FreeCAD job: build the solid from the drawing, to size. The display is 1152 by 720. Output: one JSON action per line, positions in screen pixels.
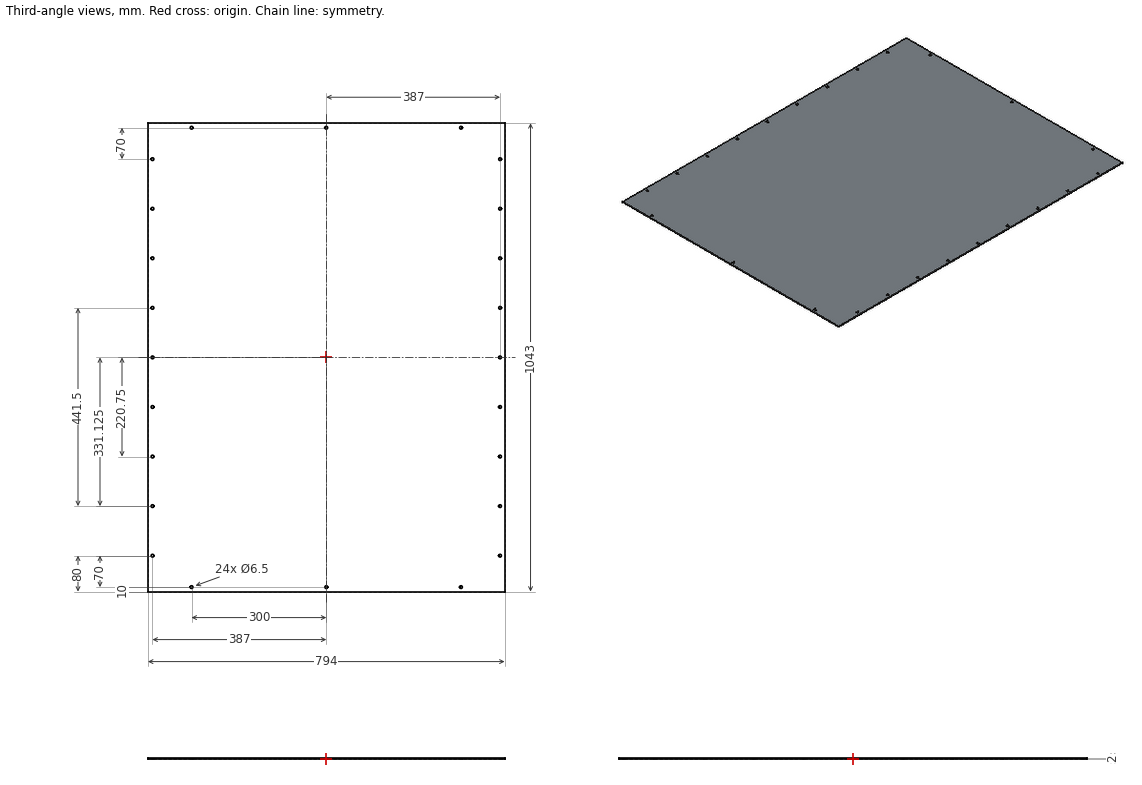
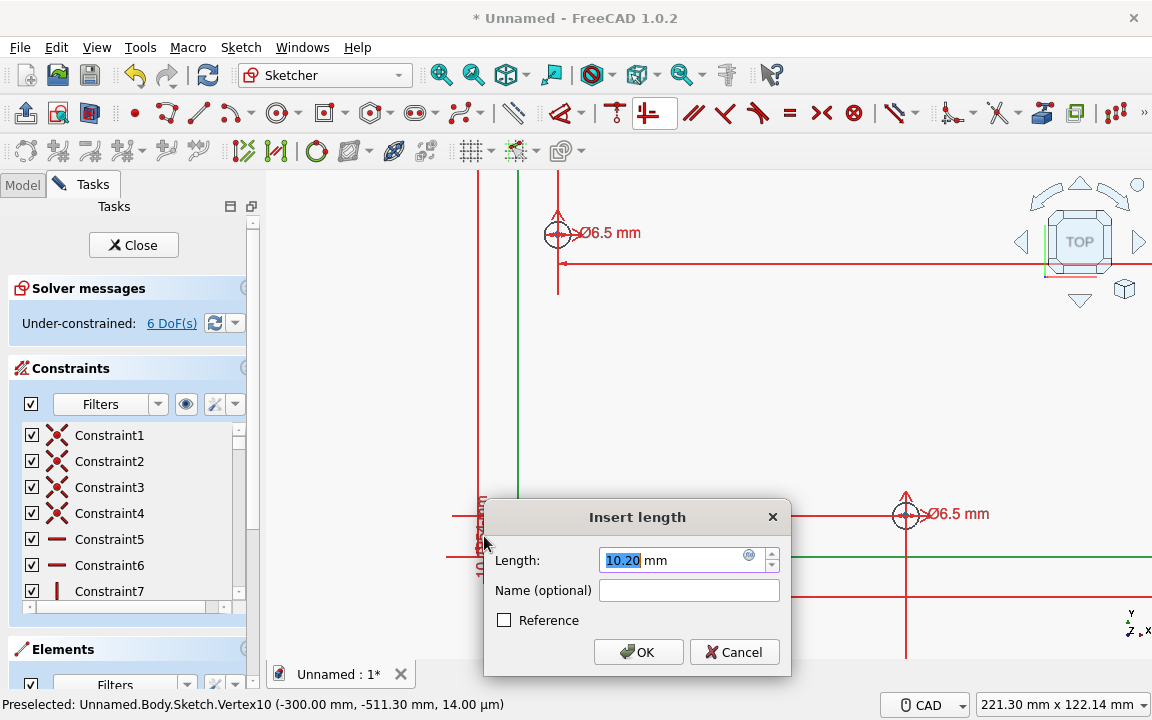
{"action": "type", "text": "10"}
{"action": "key", "text": "Return"}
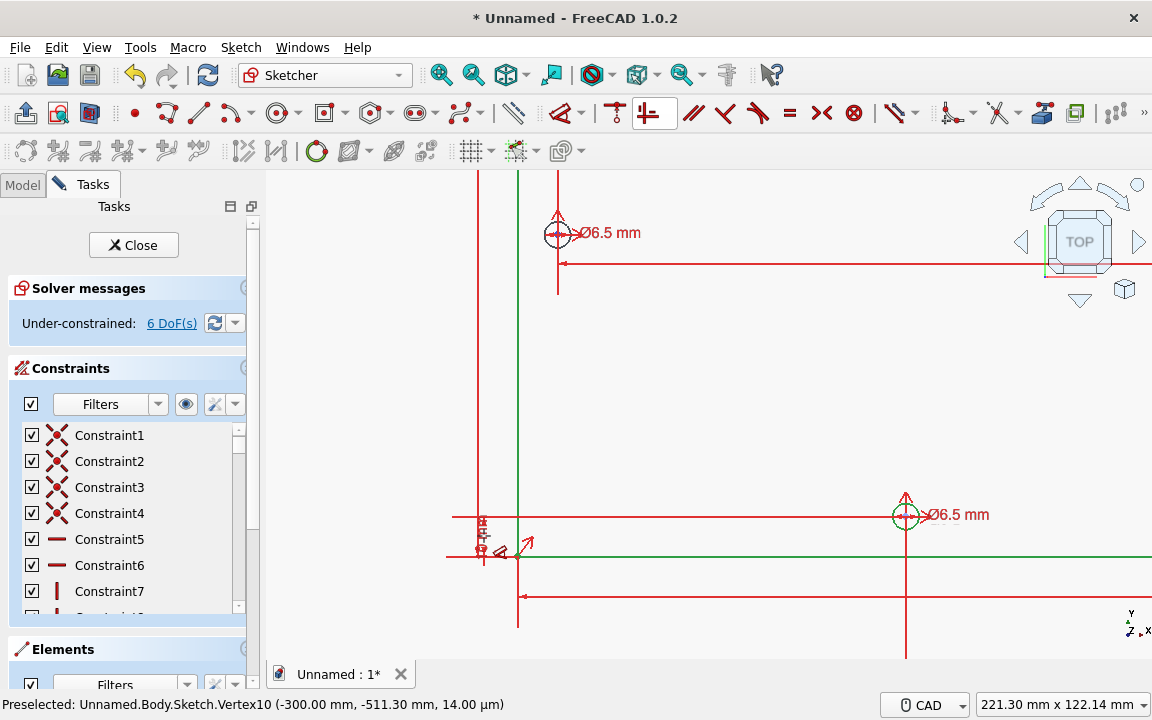
{"action": "scroll", "coordinate": [523, 571], "scroll_direction": "down", "scroll_amount": 13}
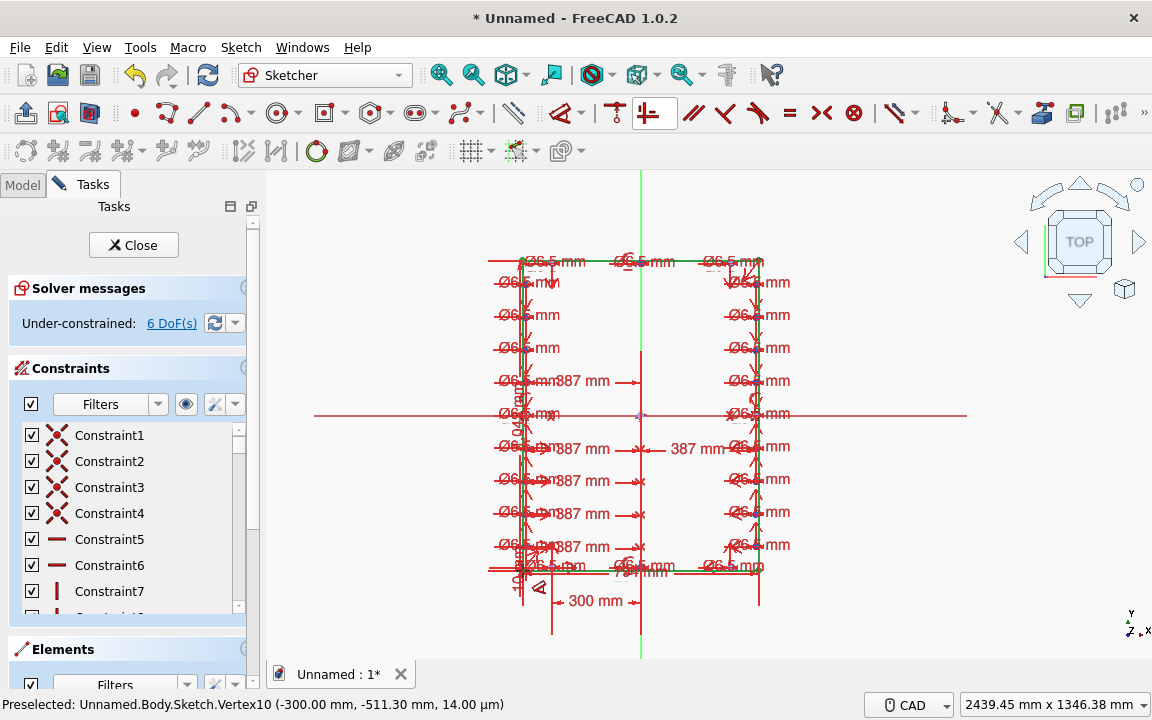
{"action": "scroll", "coordinate": [523, 571], "scroll_direction": "up", "scroll_amount": 3}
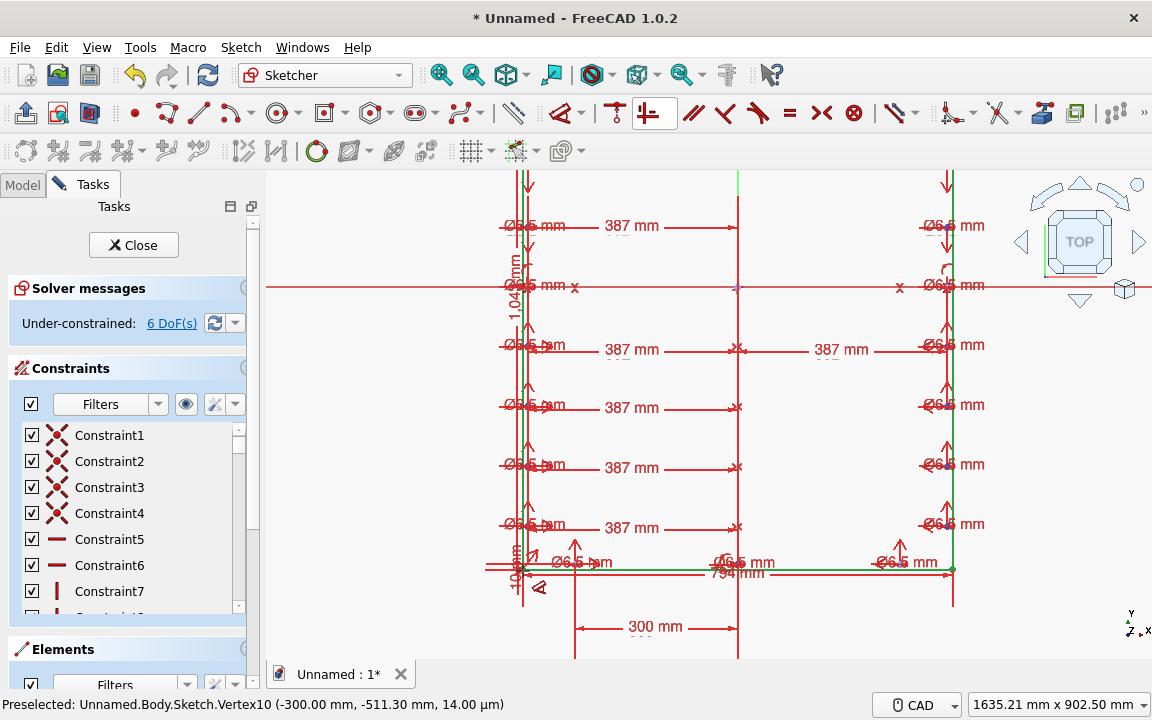
{"action": "left_click", "coordinate": [523, 570]}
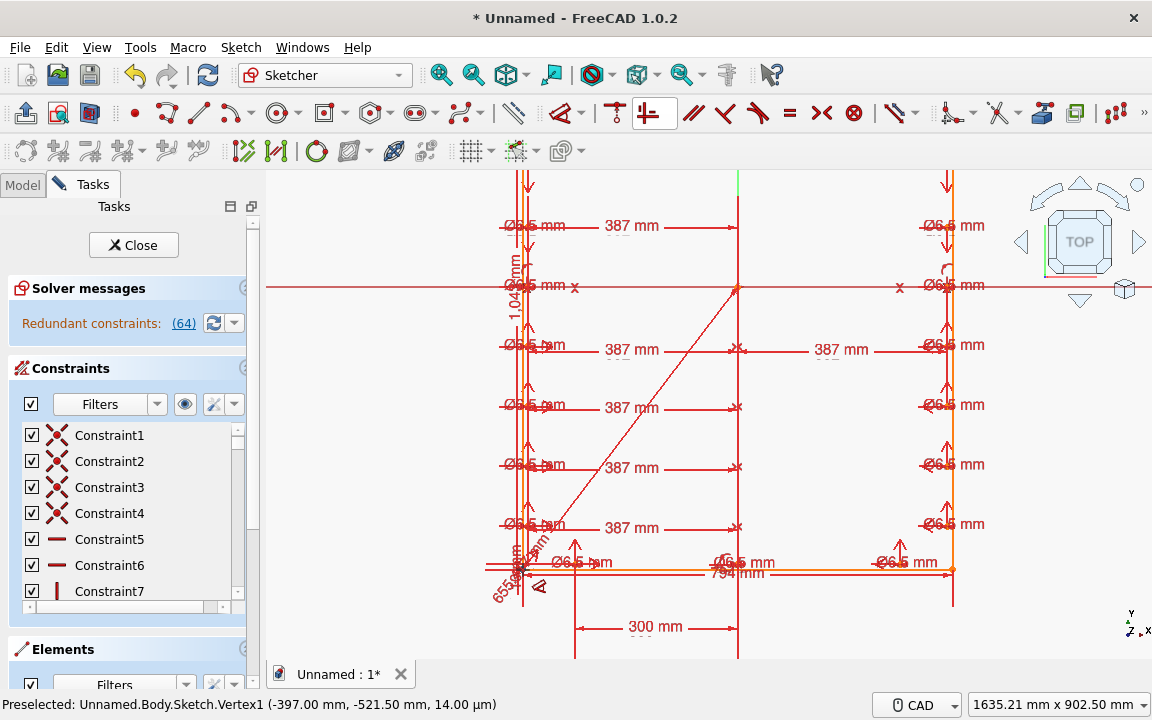
{"action": "left_click", "coordinate": [528, 526]}
{"action": "left_click", "coordinate": [489, 538]}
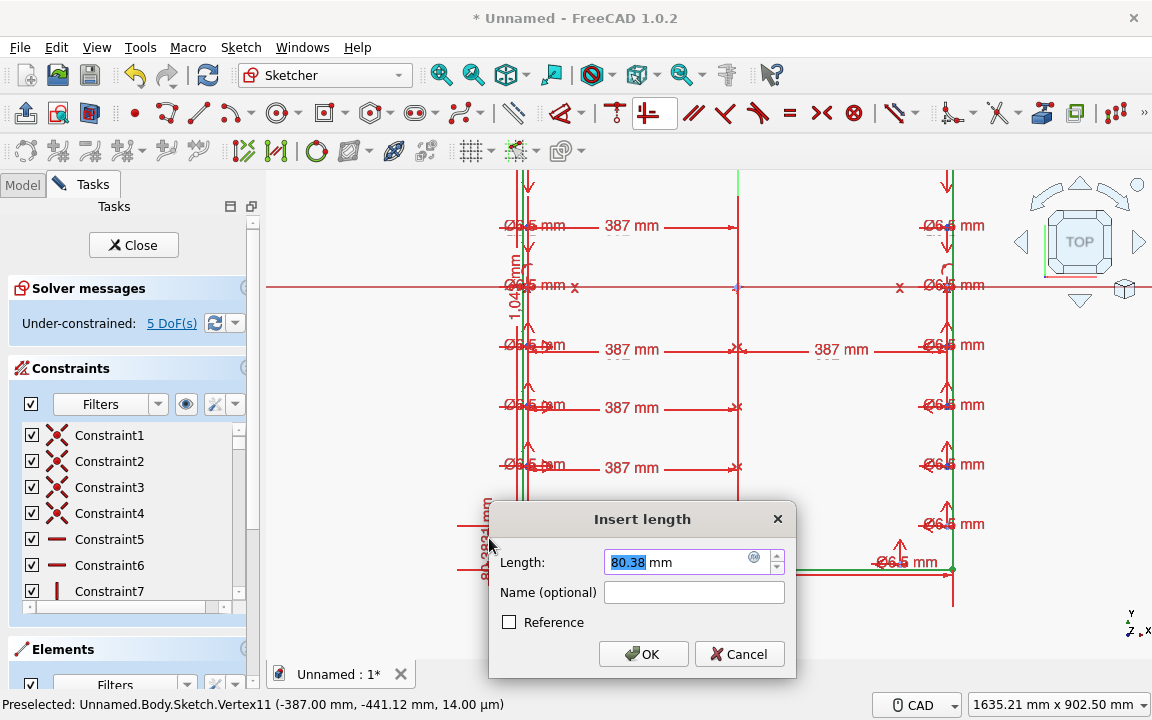
{"action": "type", "text": "80"}
{"action": "key", "text": "Return"}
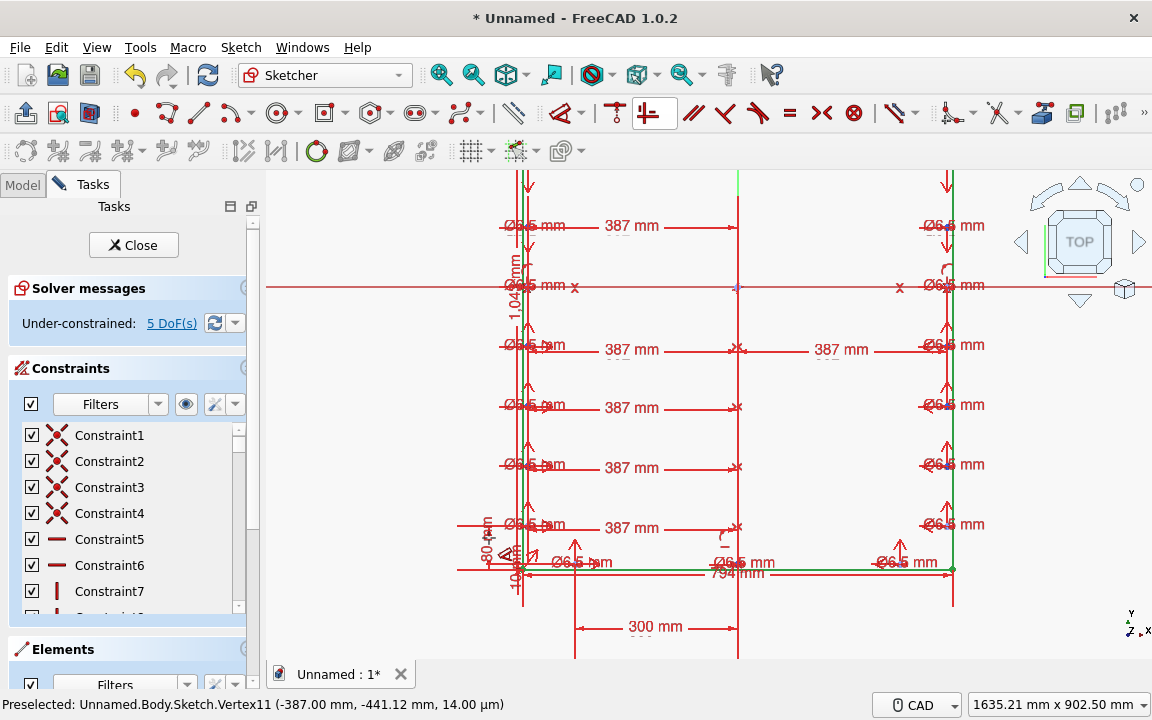
{"action": "left_click", "coordinate": [528, 526]}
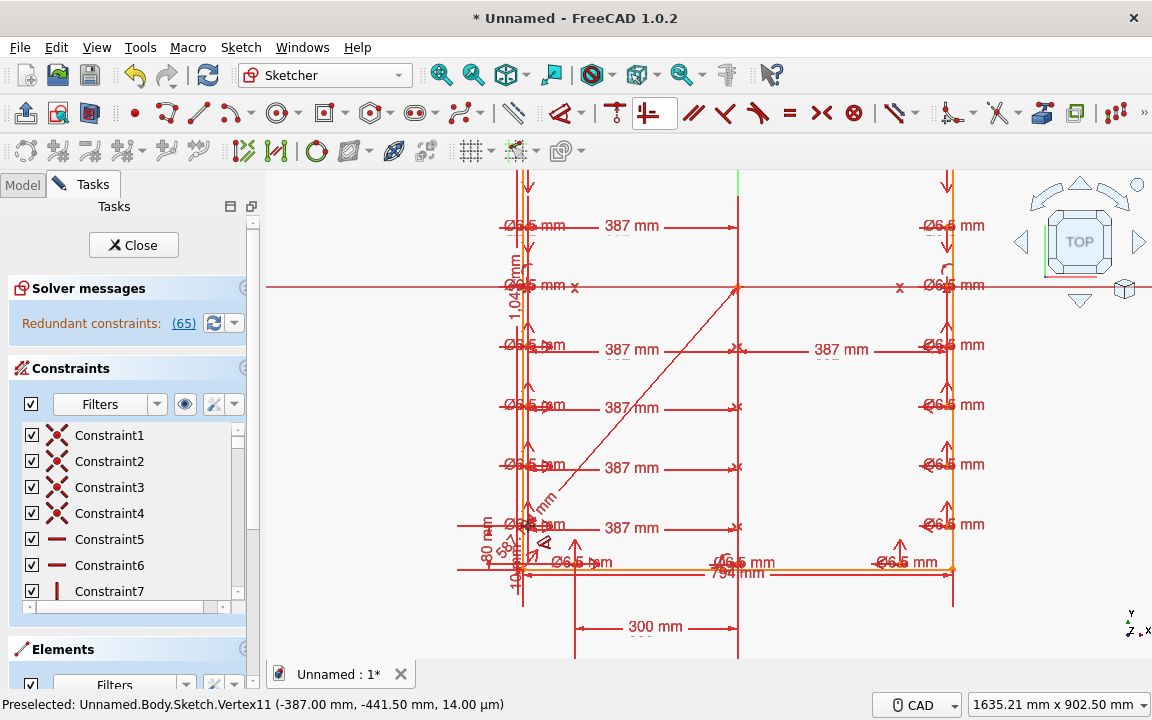
{"action": "left_click", "coordinate": [738, 565]}
{"action": "left_click", "coordinate": [772, 545]}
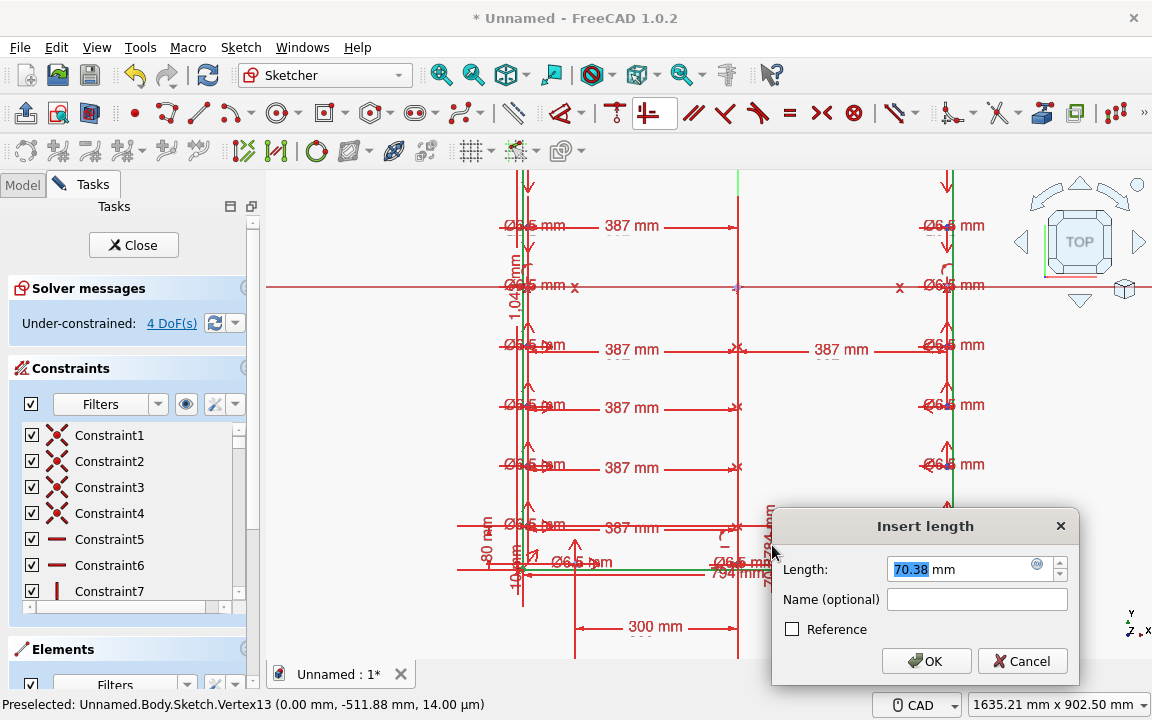
{"action": "type", "text": "70"}
{"action": "key", "text": "Return"}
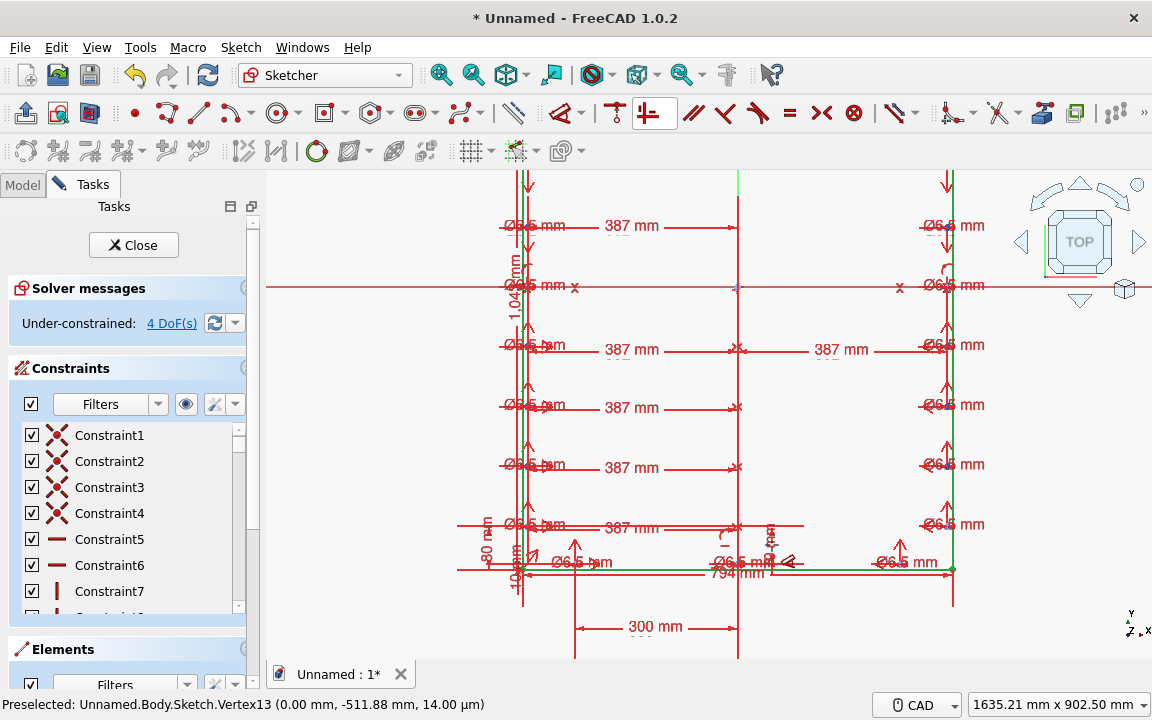
{"action": "scroll", "coordinate": [522, 569], "scroll_direction": "down", "scroll_amount": 3}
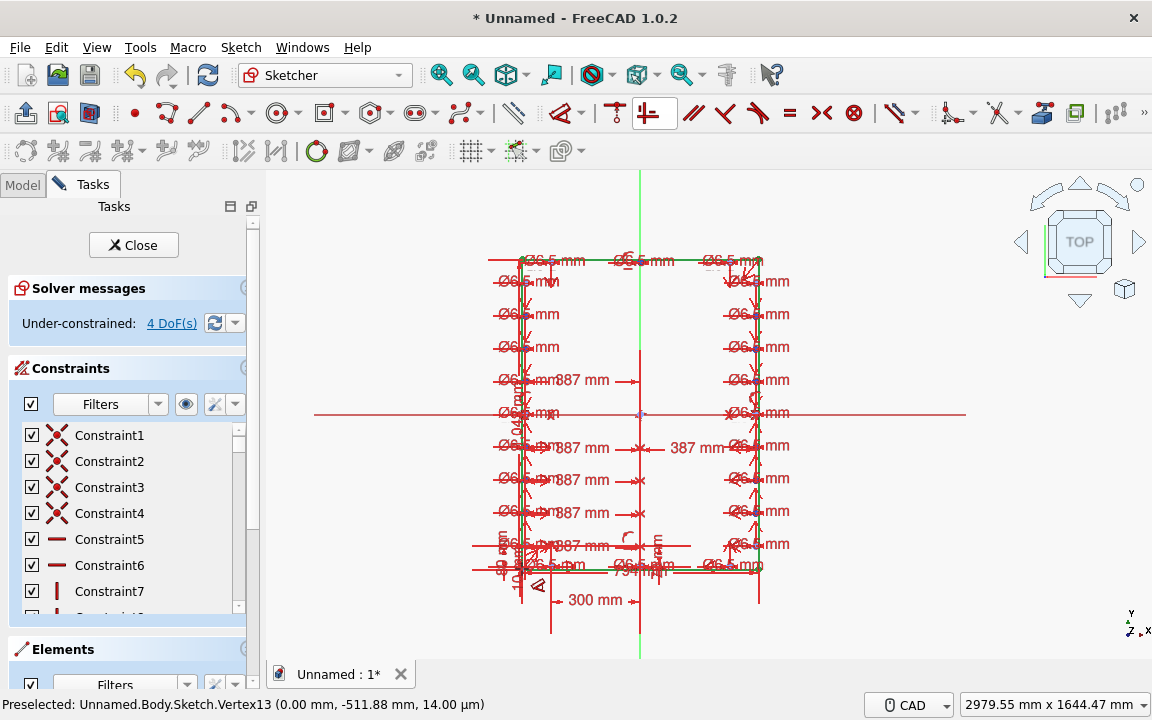
{"action": "scroll", "coordinate": [525, 283], "scroll_direction": "up", "scroll_amount": 4}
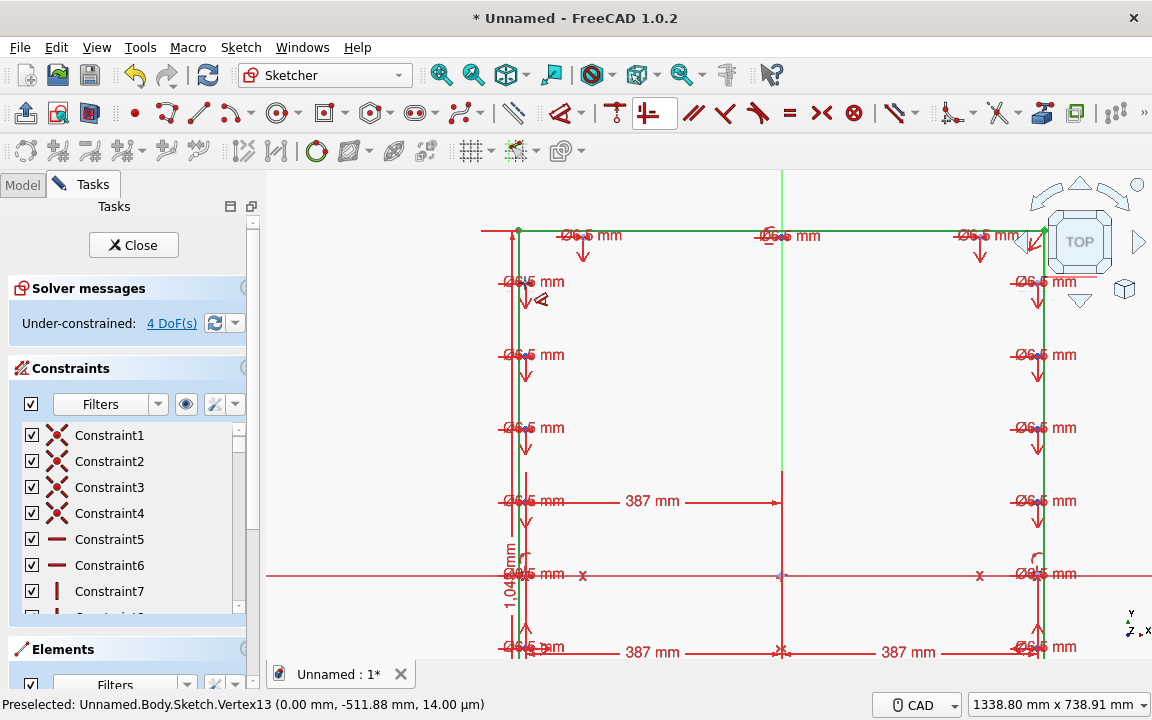
{"action": "left_click", "coordinate": [526, 284]}